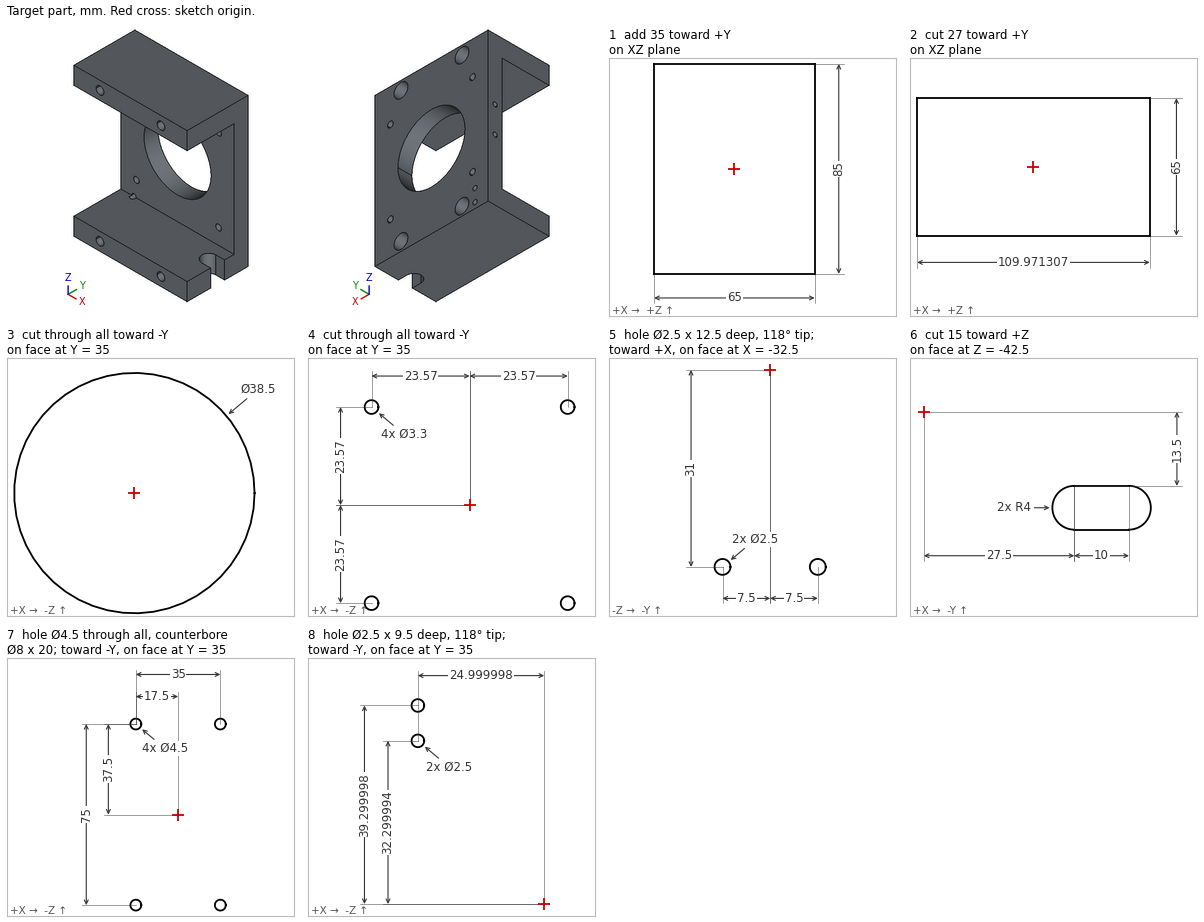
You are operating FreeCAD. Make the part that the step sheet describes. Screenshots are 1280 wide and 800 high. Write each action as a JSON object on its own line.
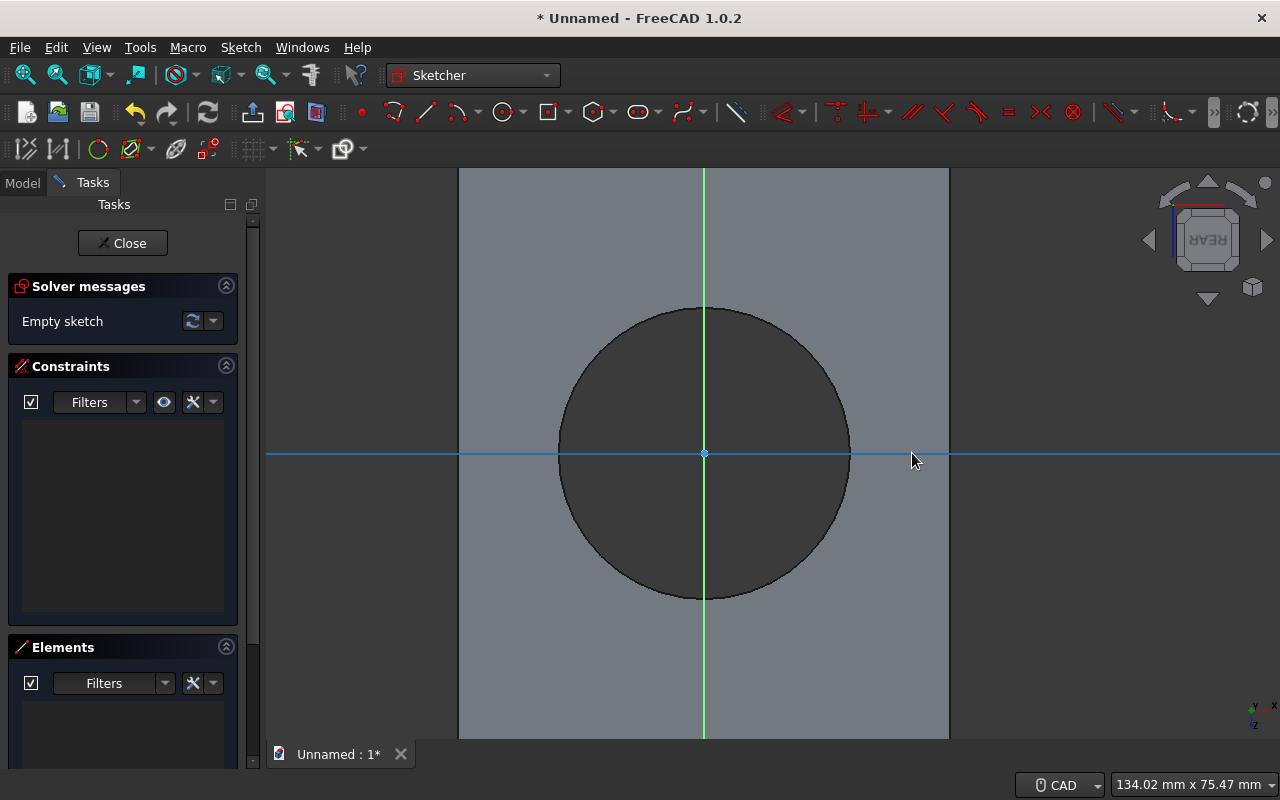
{"action": "left_click", "coordinate": [504, 112]}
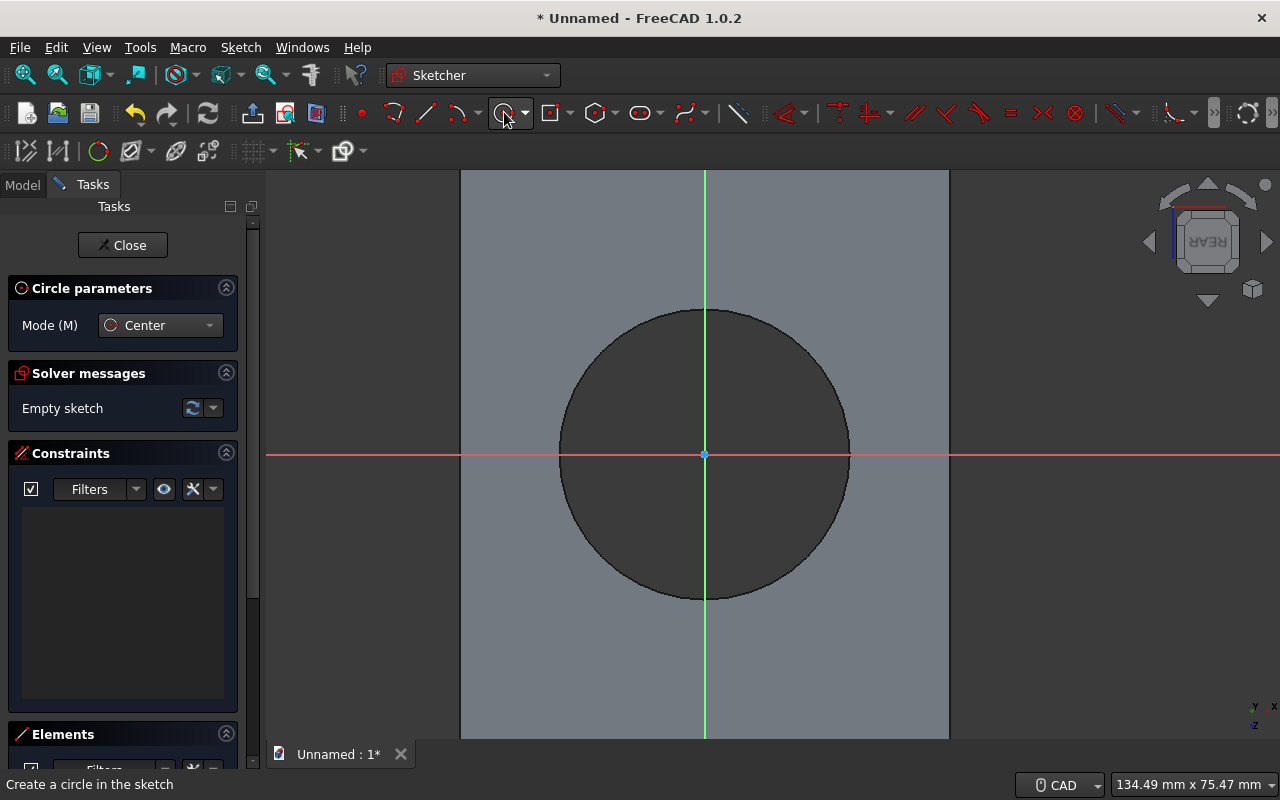
{"action": "scroll", "coordinate": [527, 277], "scroll_direction": "up", "scroll_amount": 4}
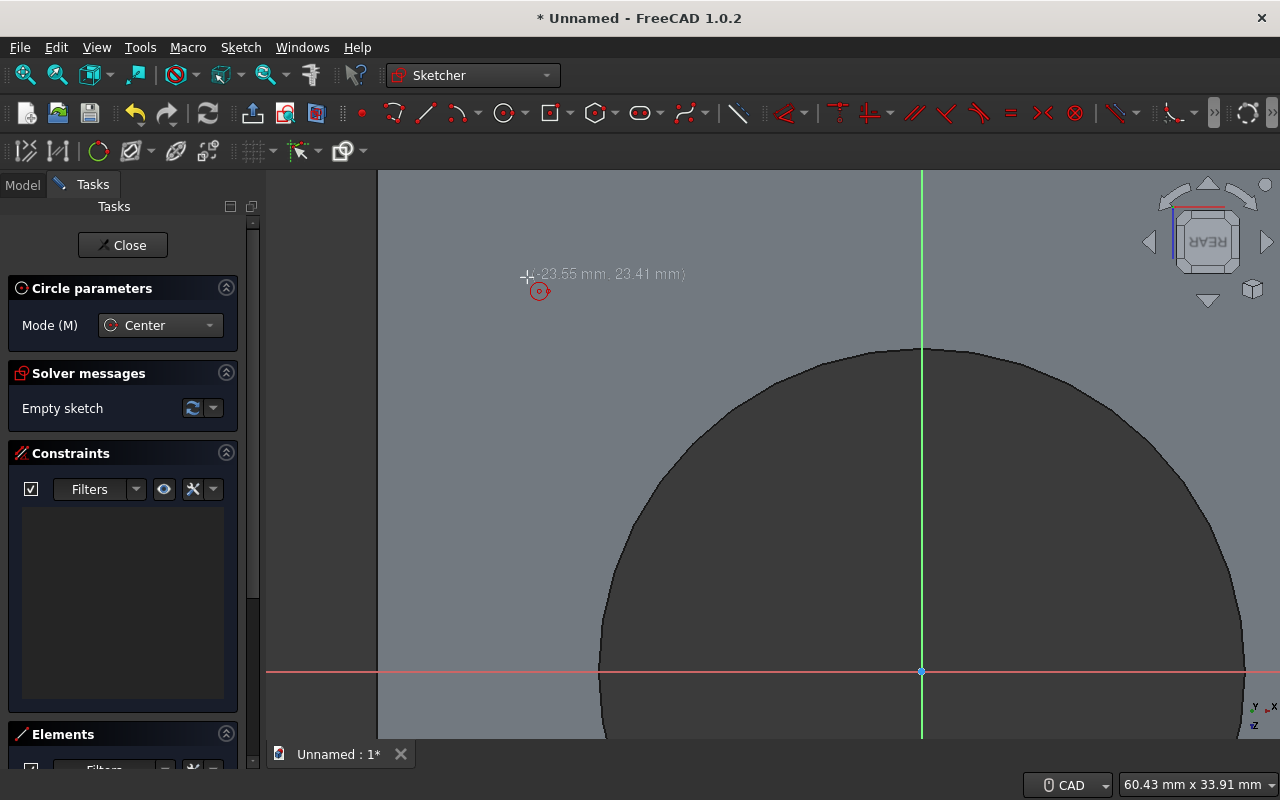
{"action": "left_click", "coordinate": [526, 276]}
{"action": "mouse_move", "coordinate": [546, 257]}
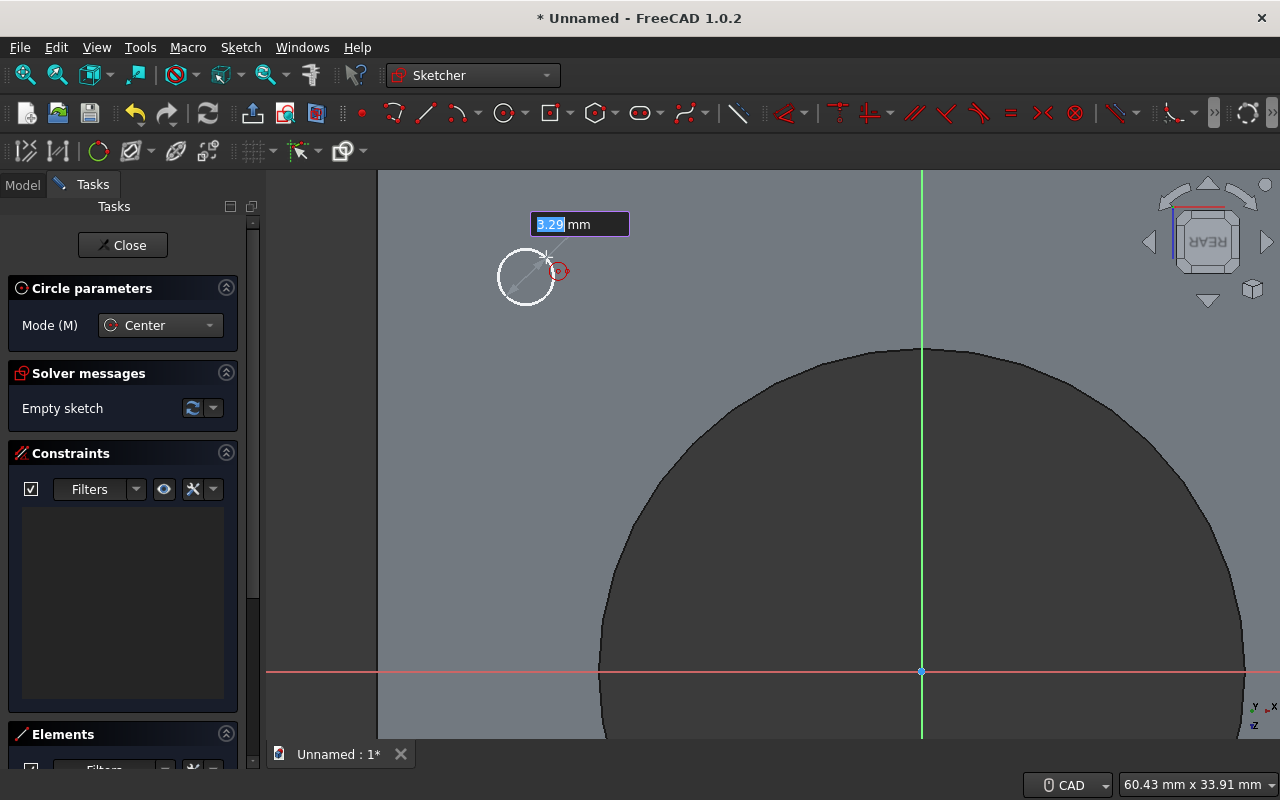
{"action": "type", "text": "3.3"}
{"action": "key", "text": "Return"}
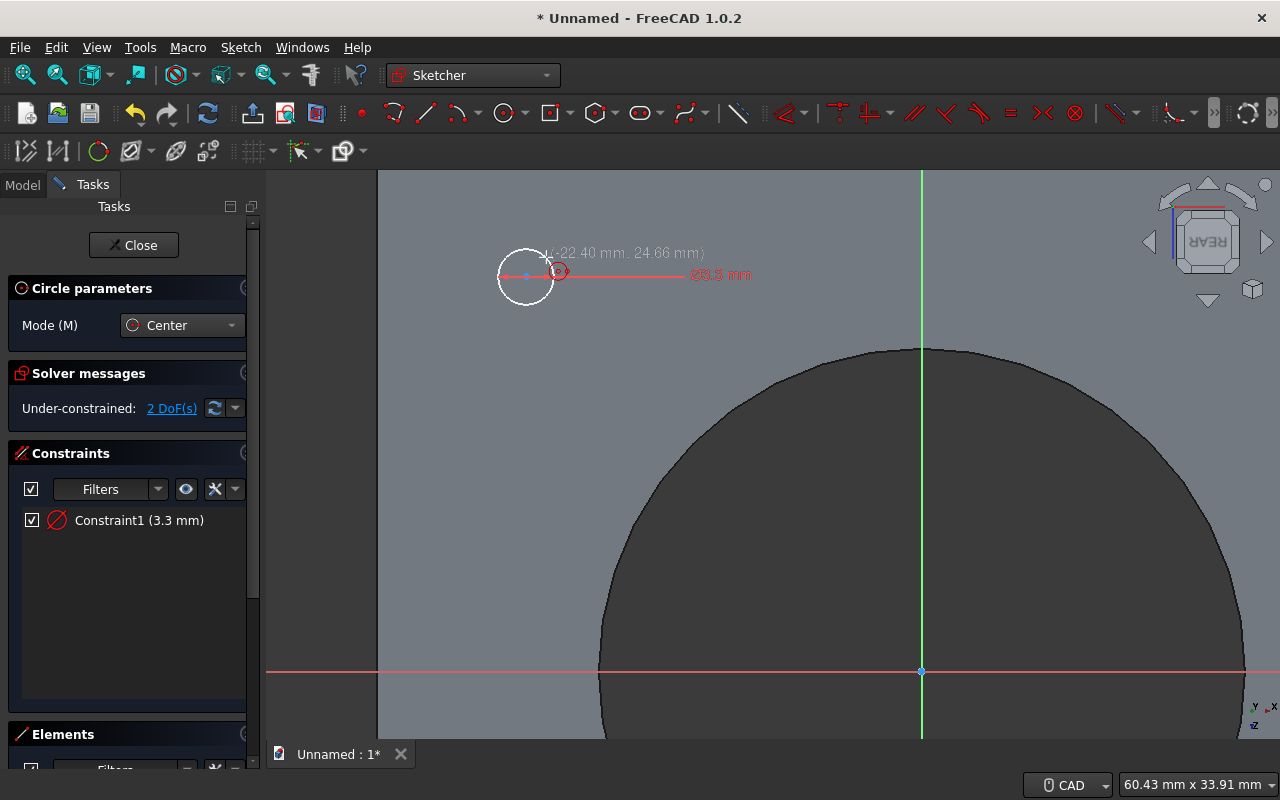
{"action": "scroll", "coordinate": [527, 277], "scroll_direction": "down", "scroll_amount": 4}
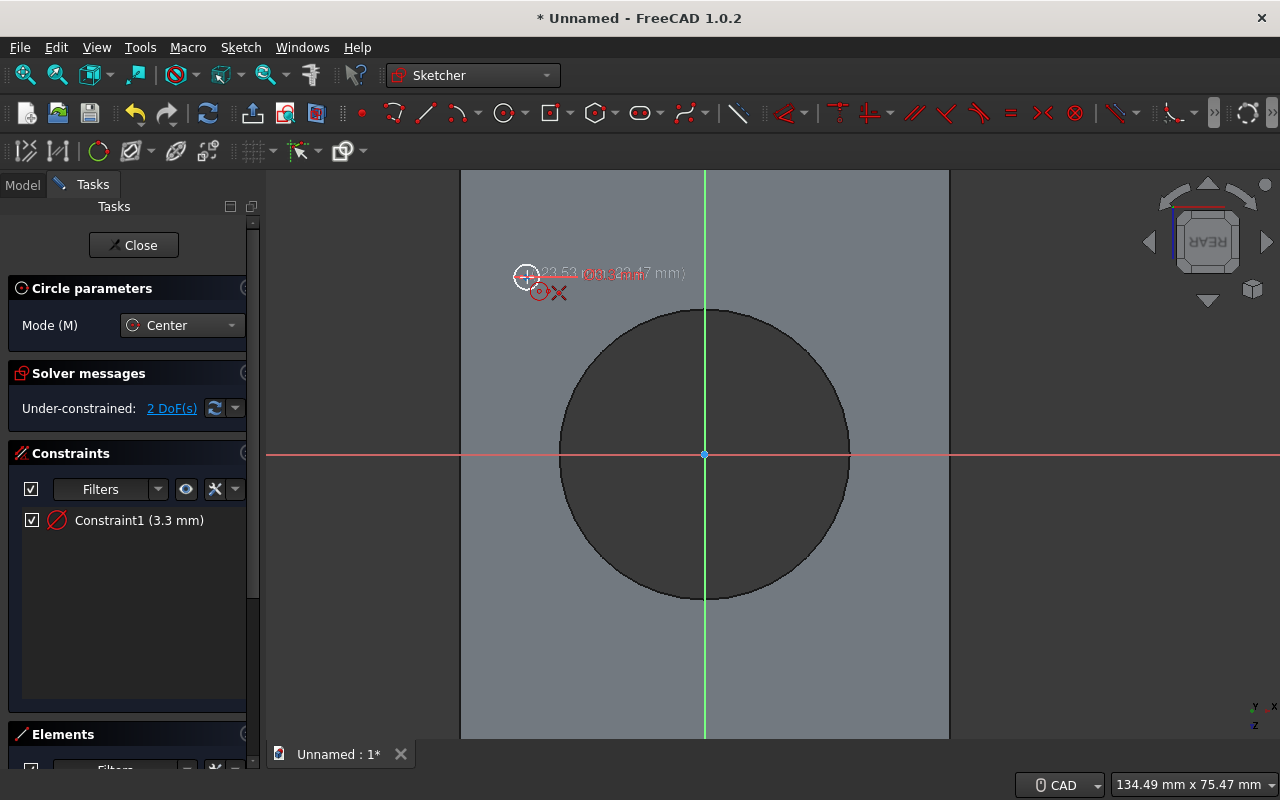
{"action": "scroll", "coordinate": [882, 277], "scroll_direction": "up", "scroll_amount": 4}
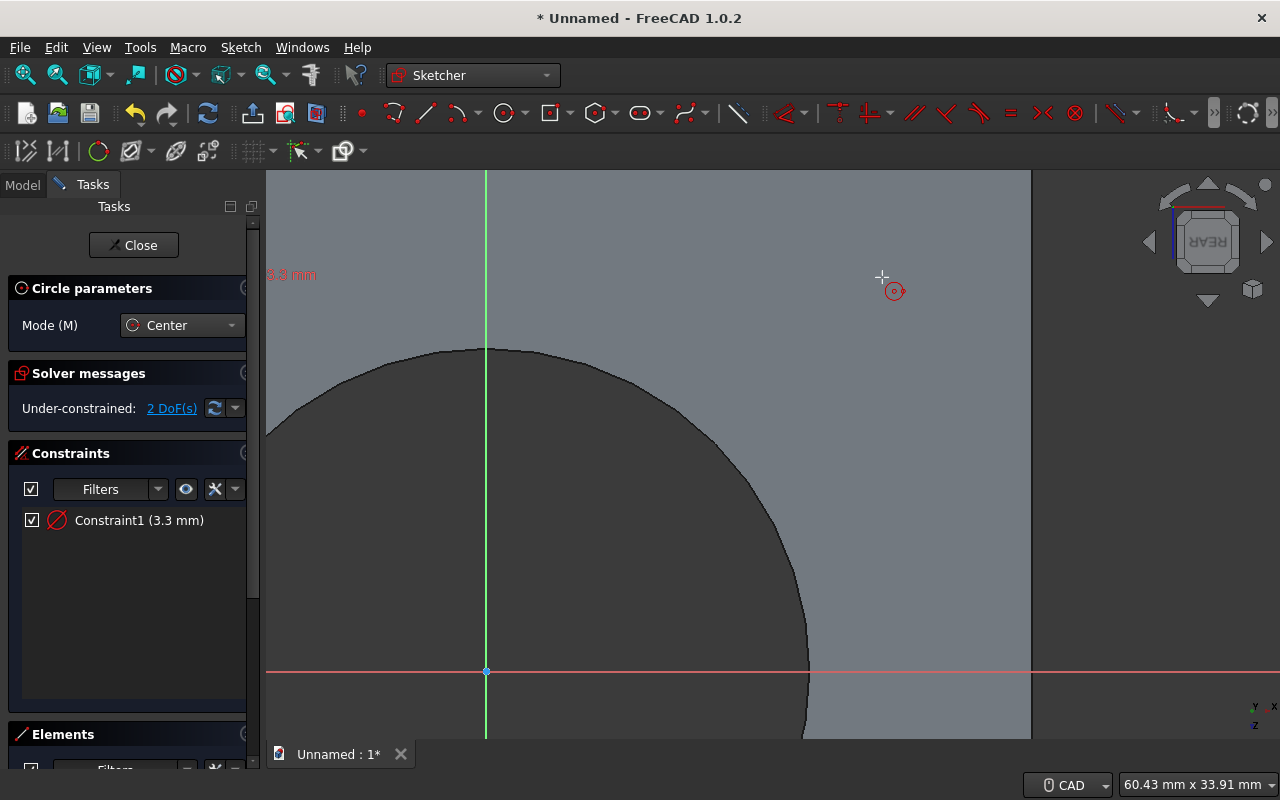
{"action": "left_click", "coordinate": [882, 276]}
{"action": "mouse_move", "coordinate": [901, 257]}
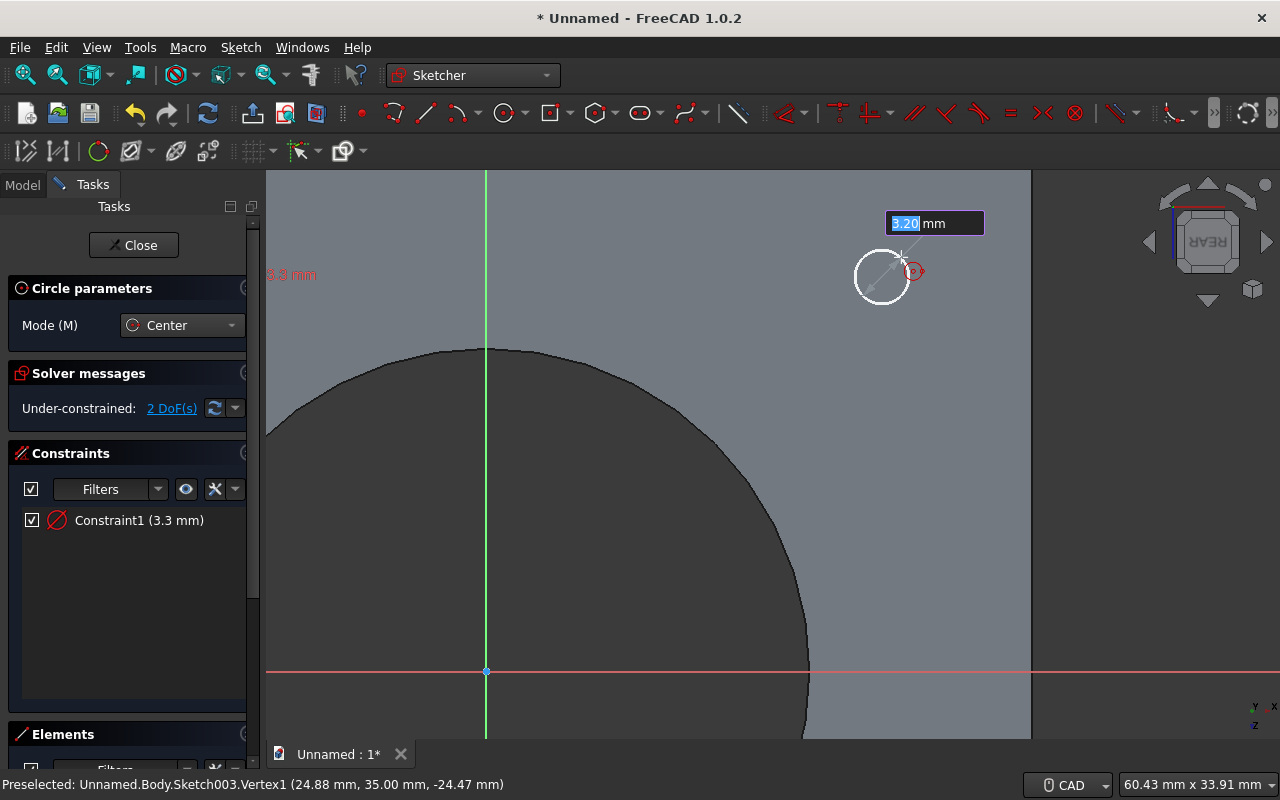
{"action": "type", "text": "3.3"}
{"action": "key", "text": "Return"}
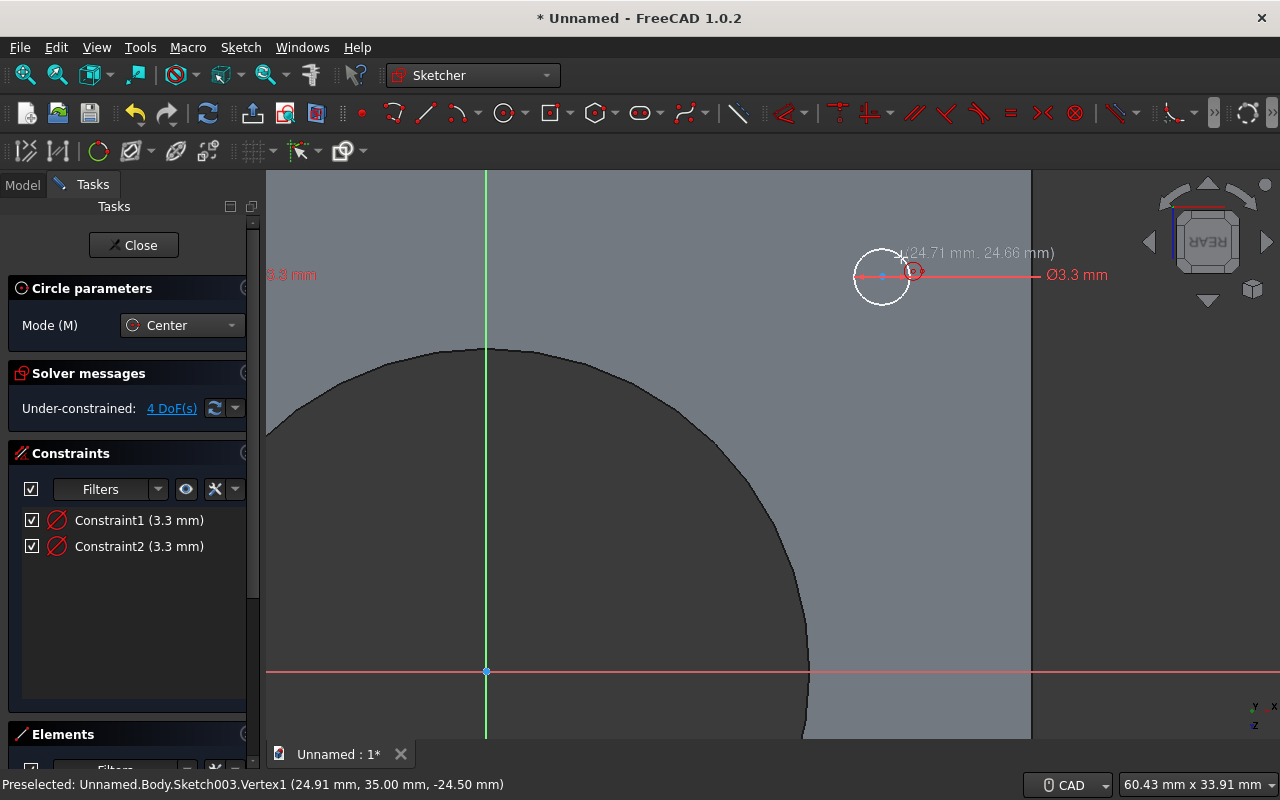
{"action": "scroll", "coordinate": [882, 277], "scroll_direction": "down", "scroll_amount": 4}